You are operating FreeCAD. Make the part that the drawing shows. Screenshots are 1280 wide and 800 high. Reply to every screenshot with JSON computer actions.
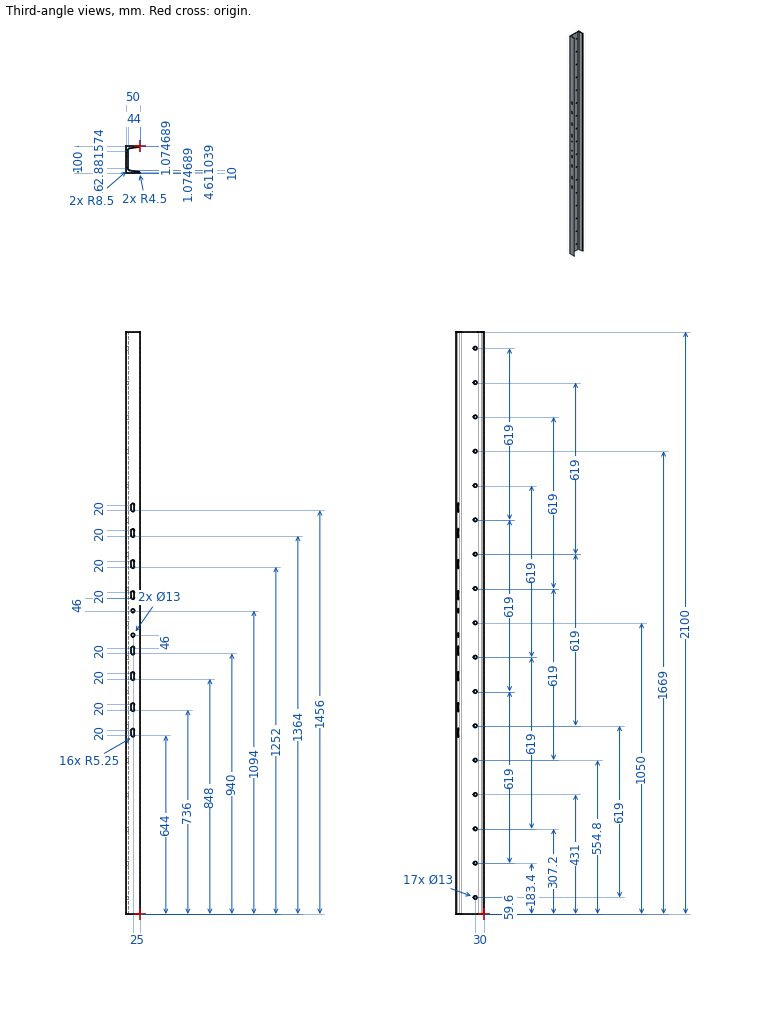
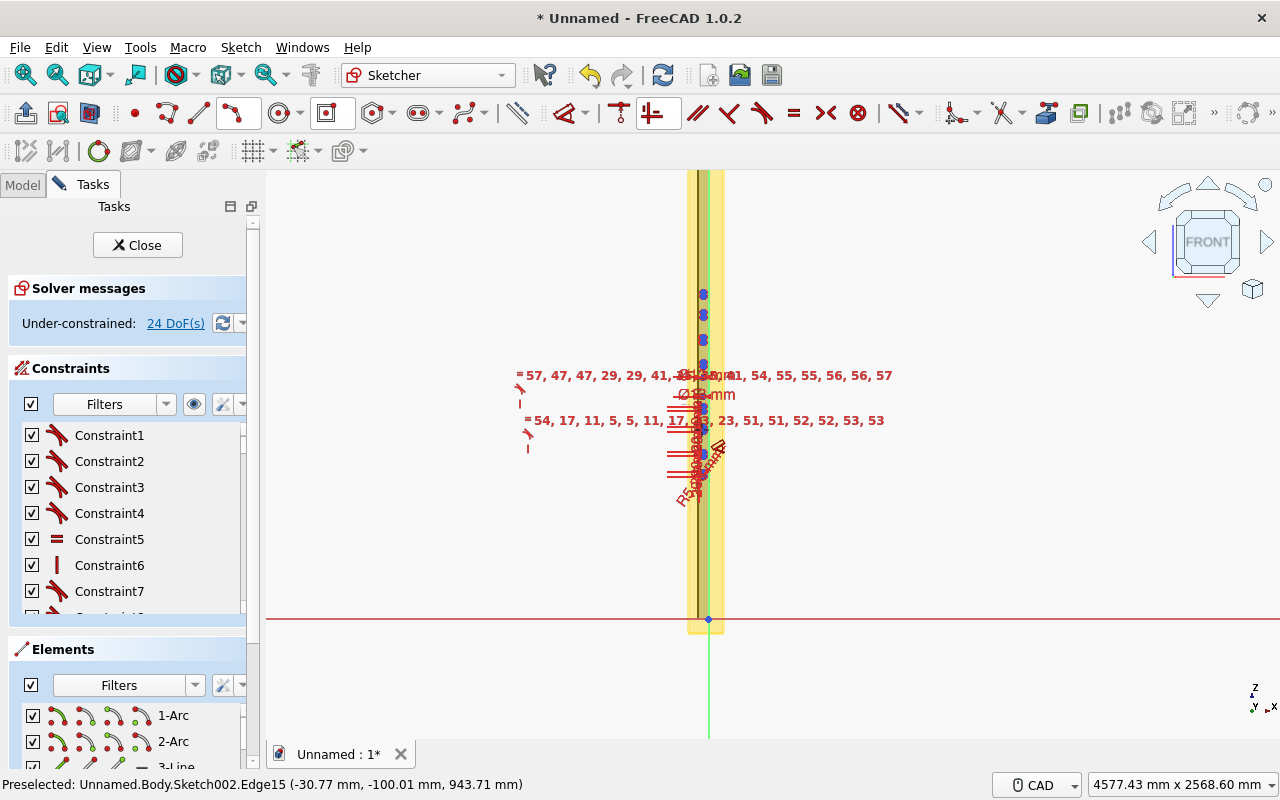
{"action": "scroll", "coordinate": [702, 341], "scroll_direction": "up", "scroll_amount": 12}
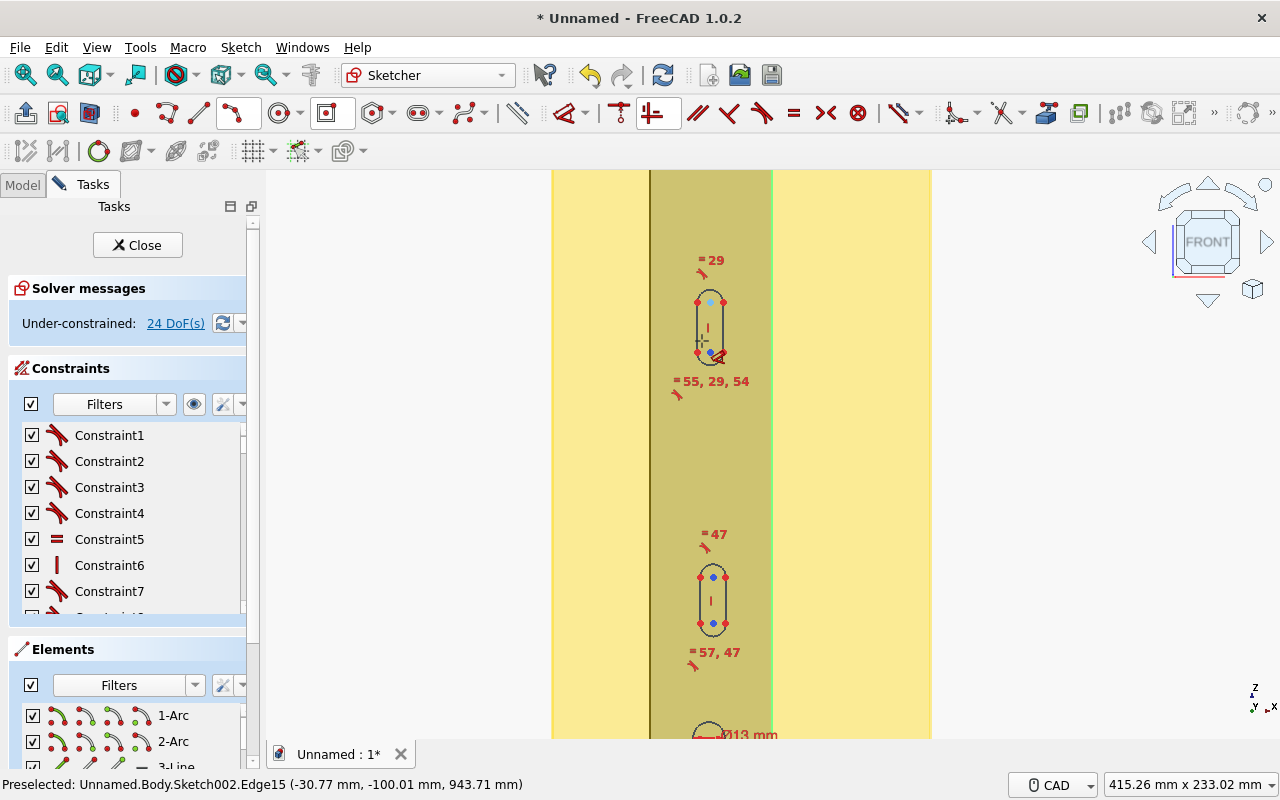
{"action": "left_click", "coordinate": [697, 338]}
{"action": "left_click", "coordinate": [663, 328]}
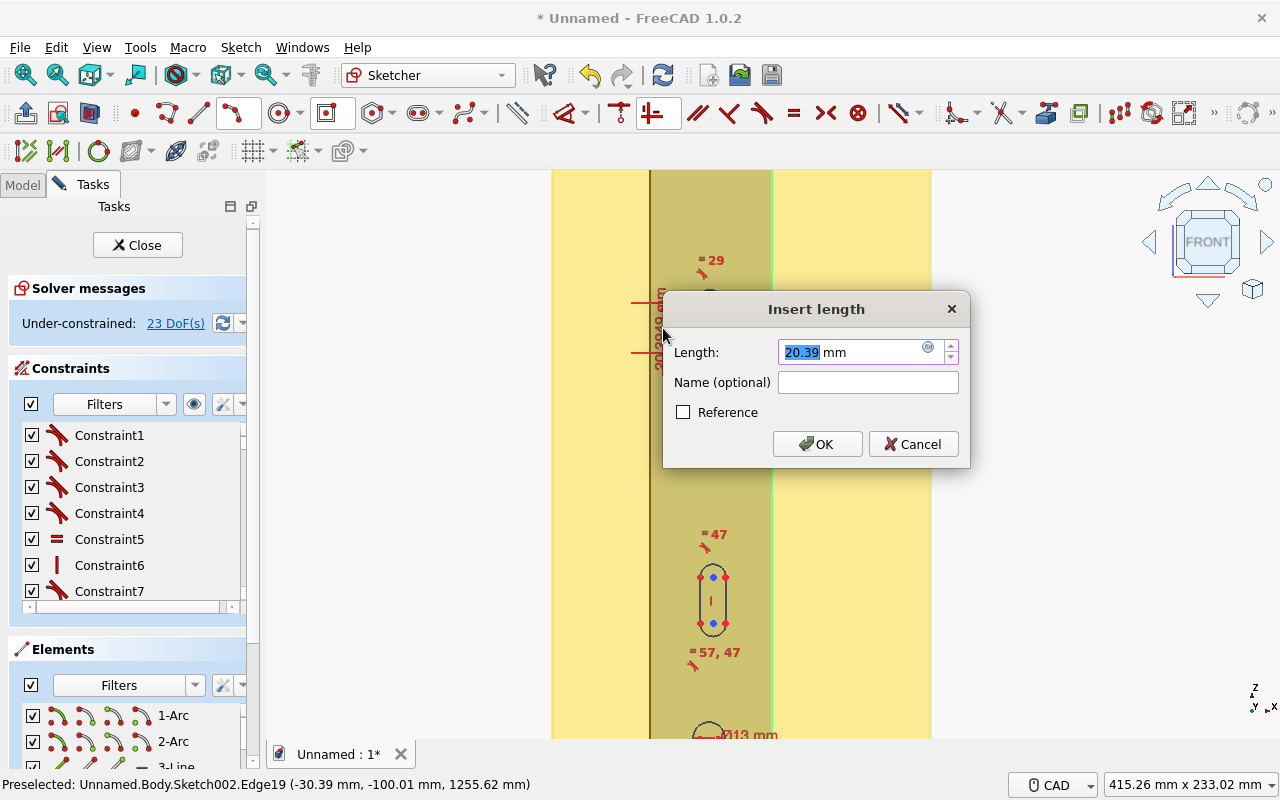
{"action": "type", "text": "20"}
{"action": "key", "text": "Return"}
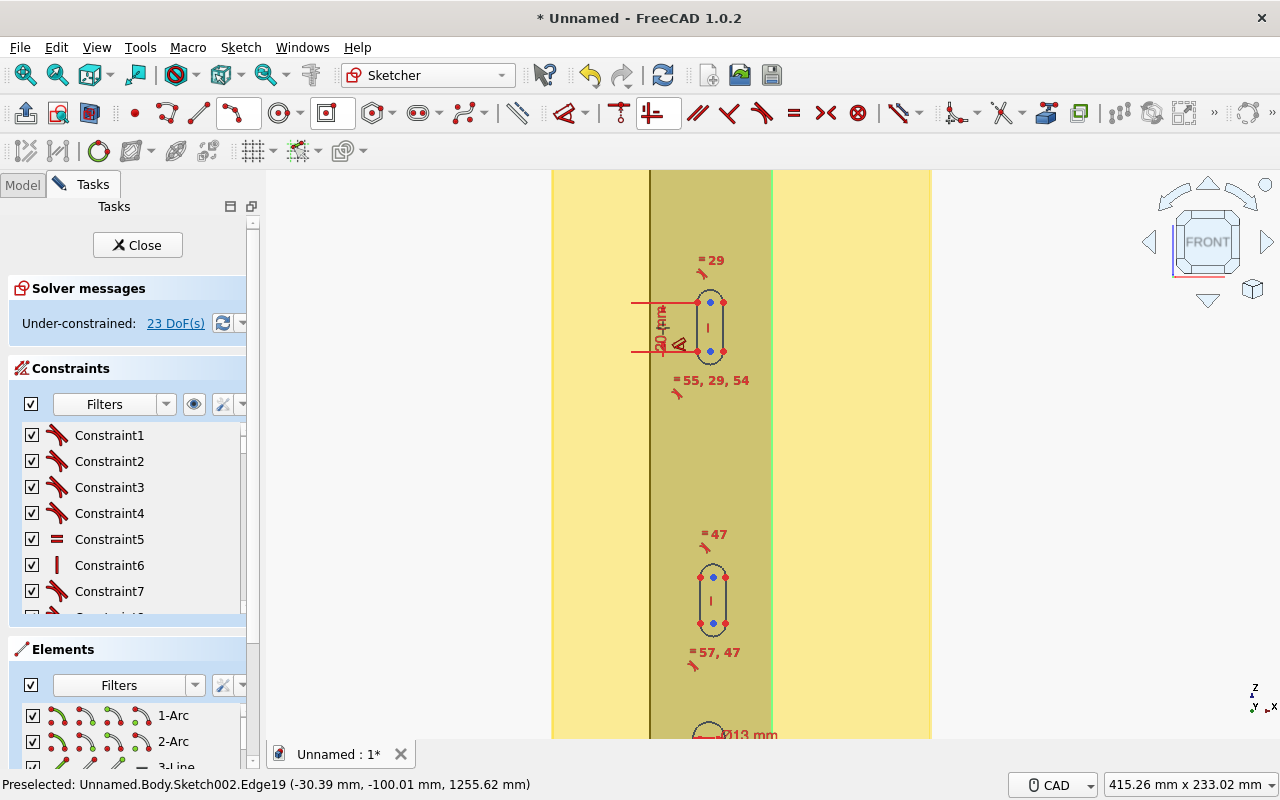
{"action": "scroll", "coordinate": [702, 341], "scroll_direction": "down", "scroll_amount": 12}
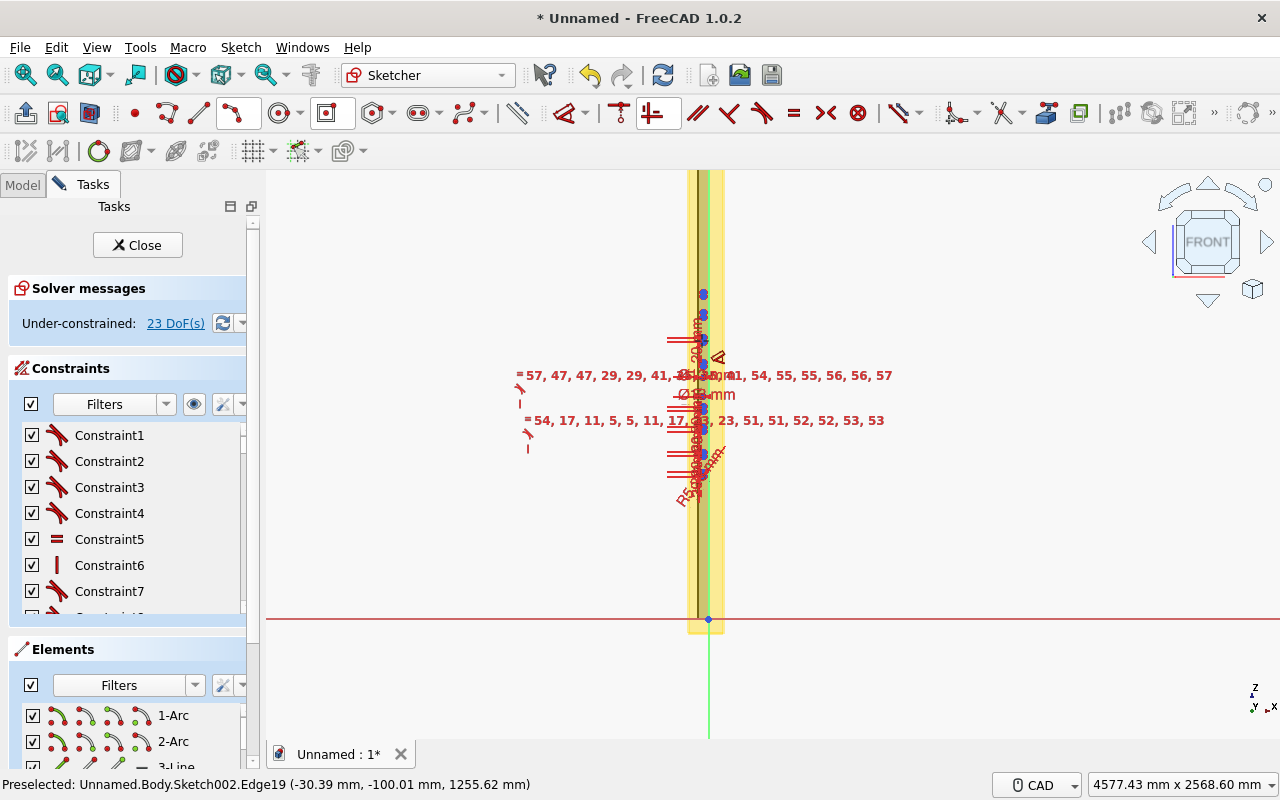
{"action": "scroll", "coordinate": [702, 296], "scroll_direction": "up", "scroll_amount": 12}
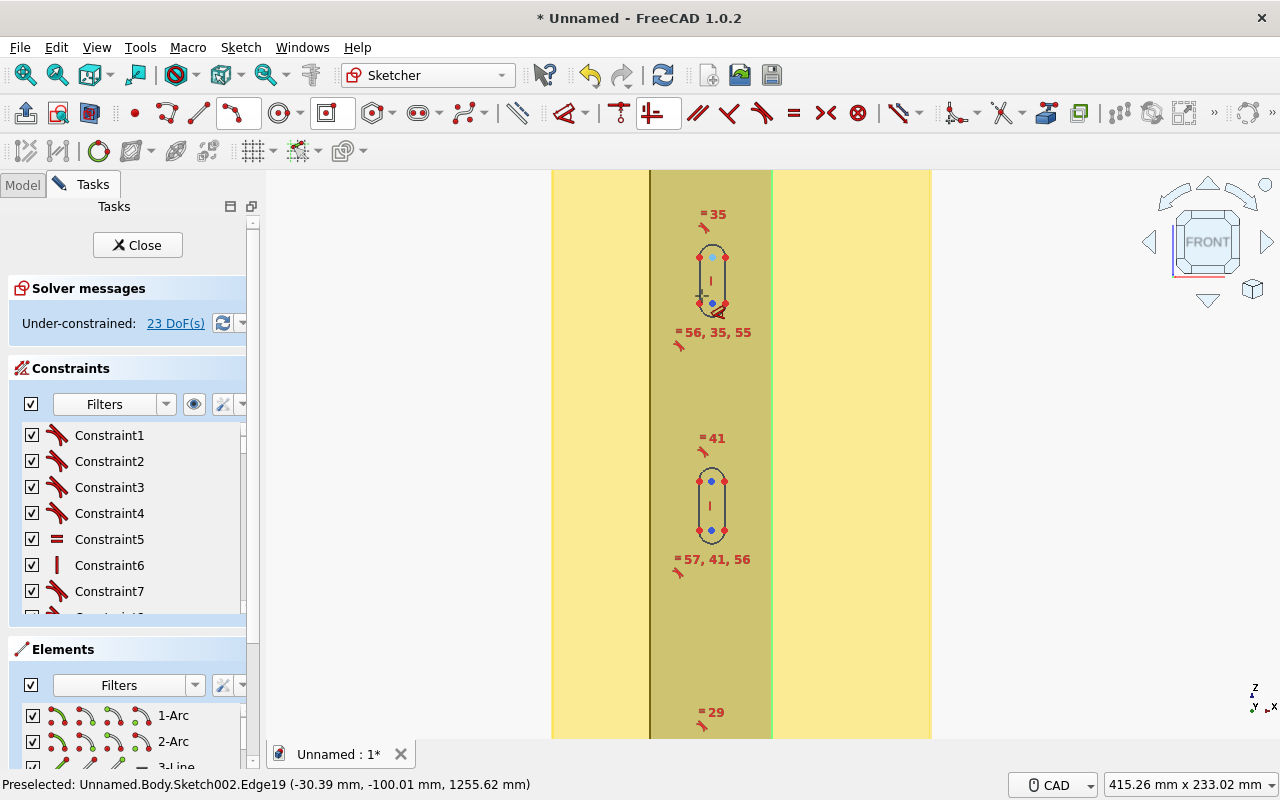
{"action": "left_click", "coordinate": [700, 290]}
{"action": "left_click", "coordinate": [666, 281]}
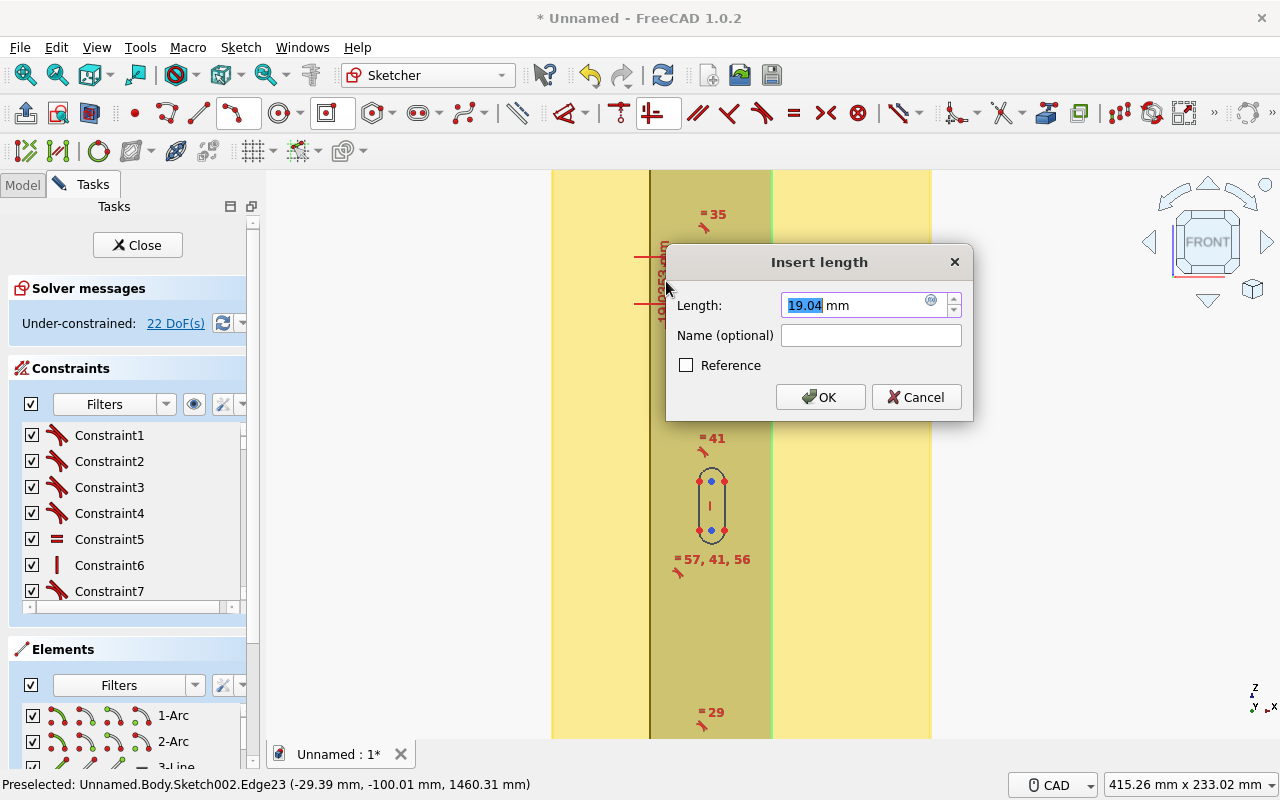
{"action": "type", "text": "20"}
{"action": "key", "text": "Return"}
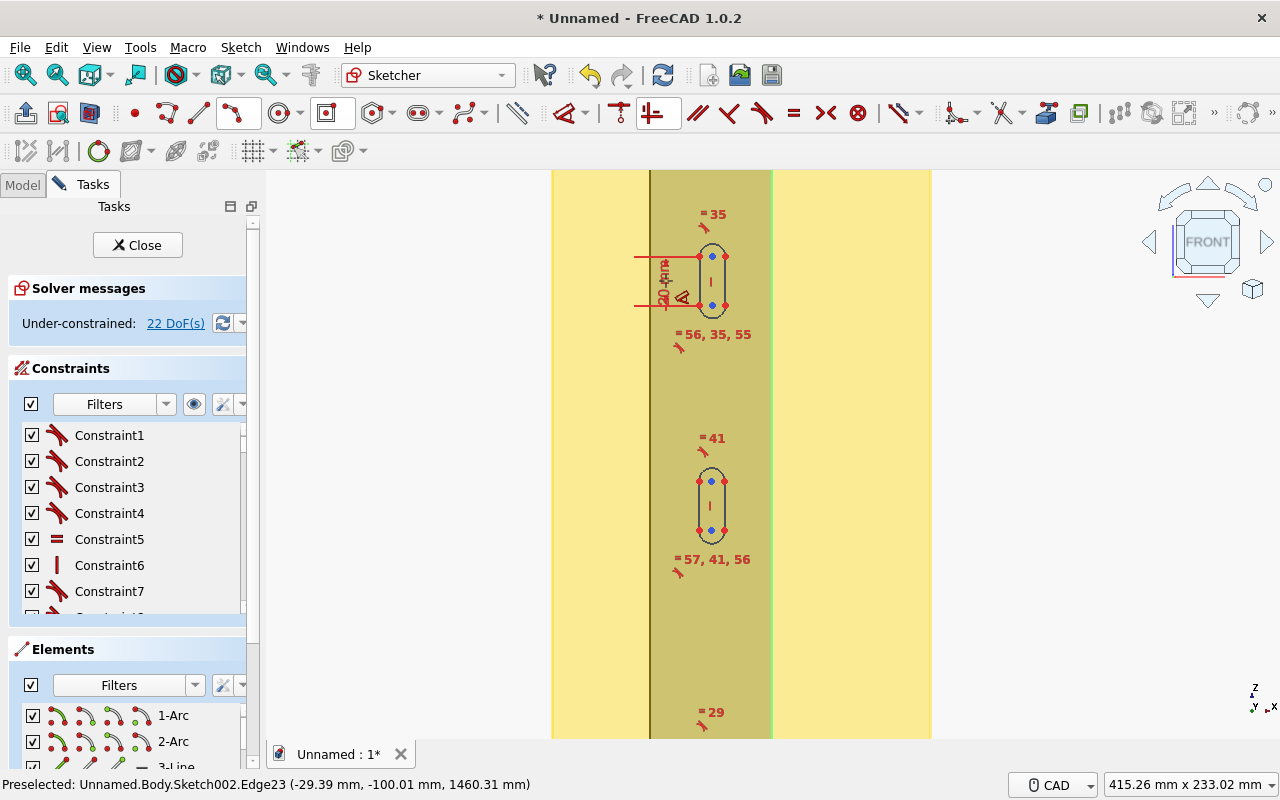
{"action": "left_click", "coordinate": [699, 516]}
{"action": "left_click", "coordinate": [665, 506]}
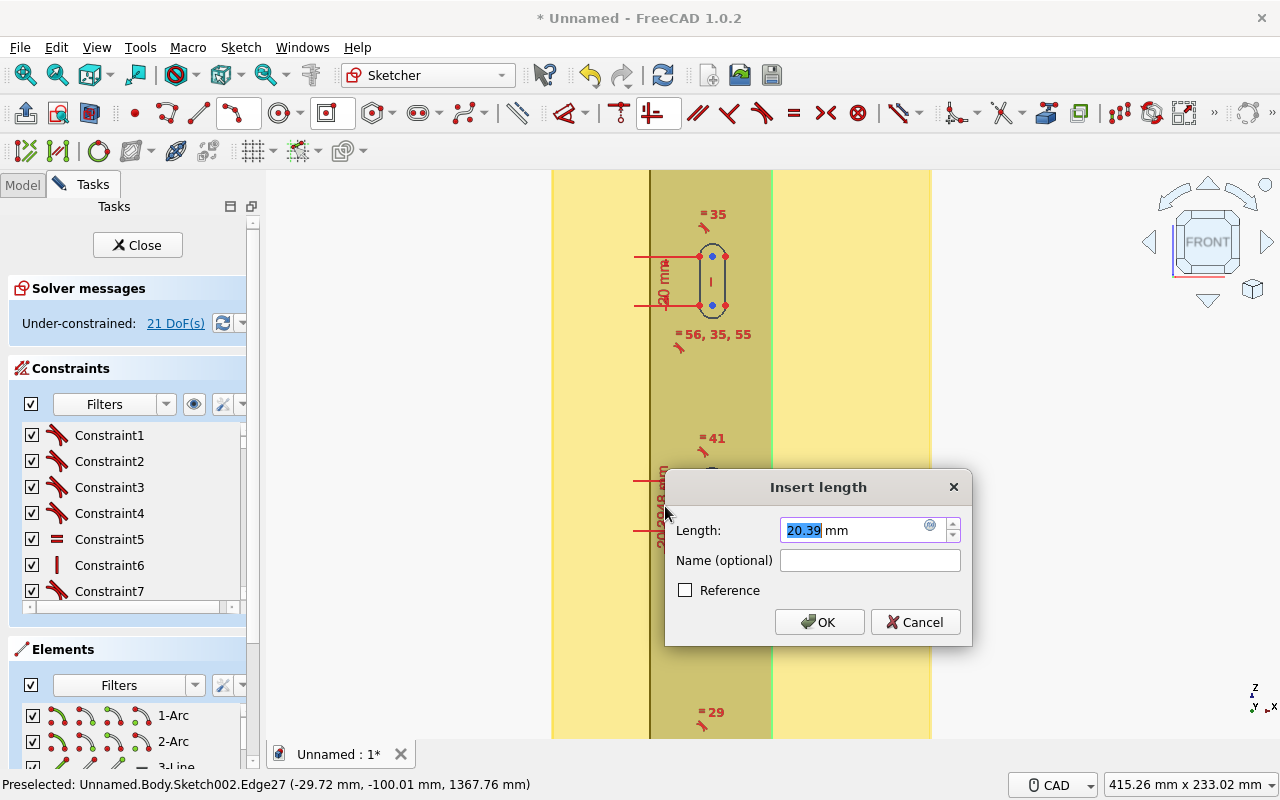
{"action": "type", "text": "20"}
{"action": "key", "text": "Return"}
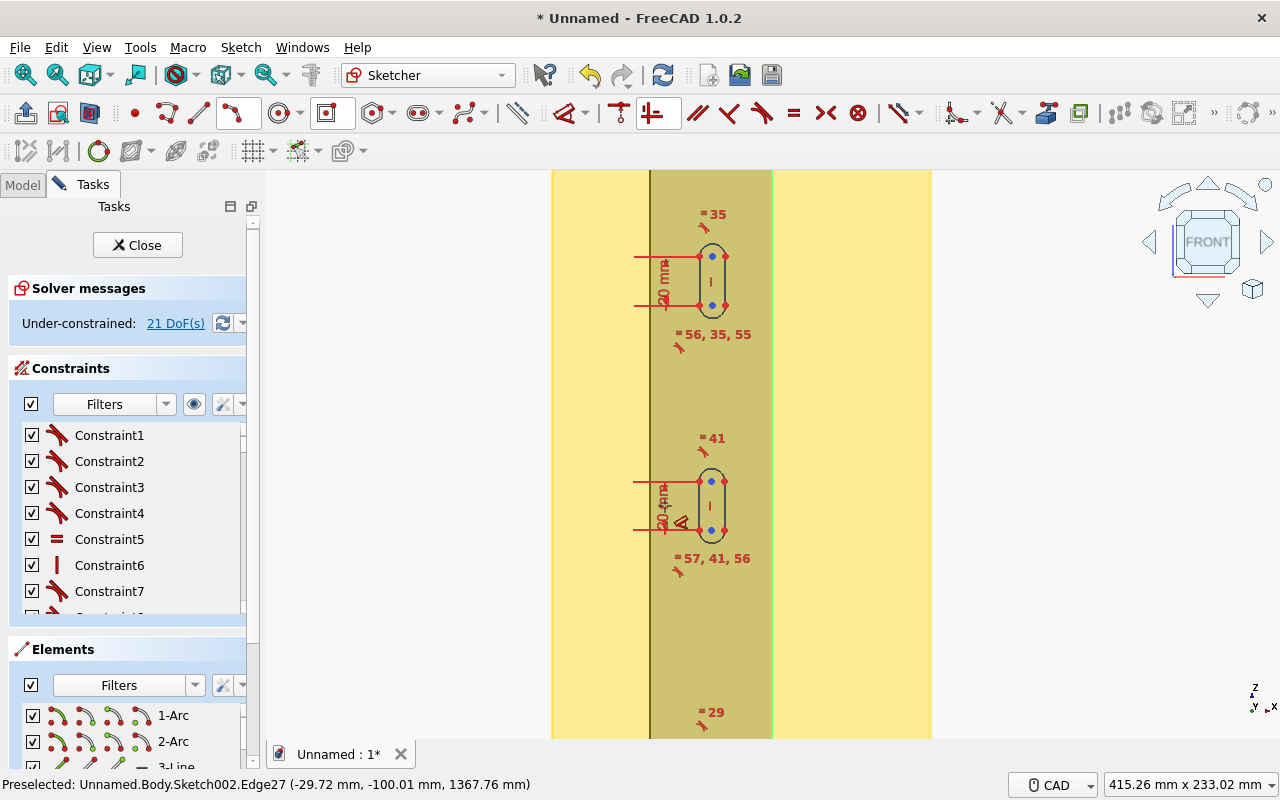
{"action": "scroll", "coordinate": [702, 295], "scroll_direction": "down", "scroll_amount": 12}